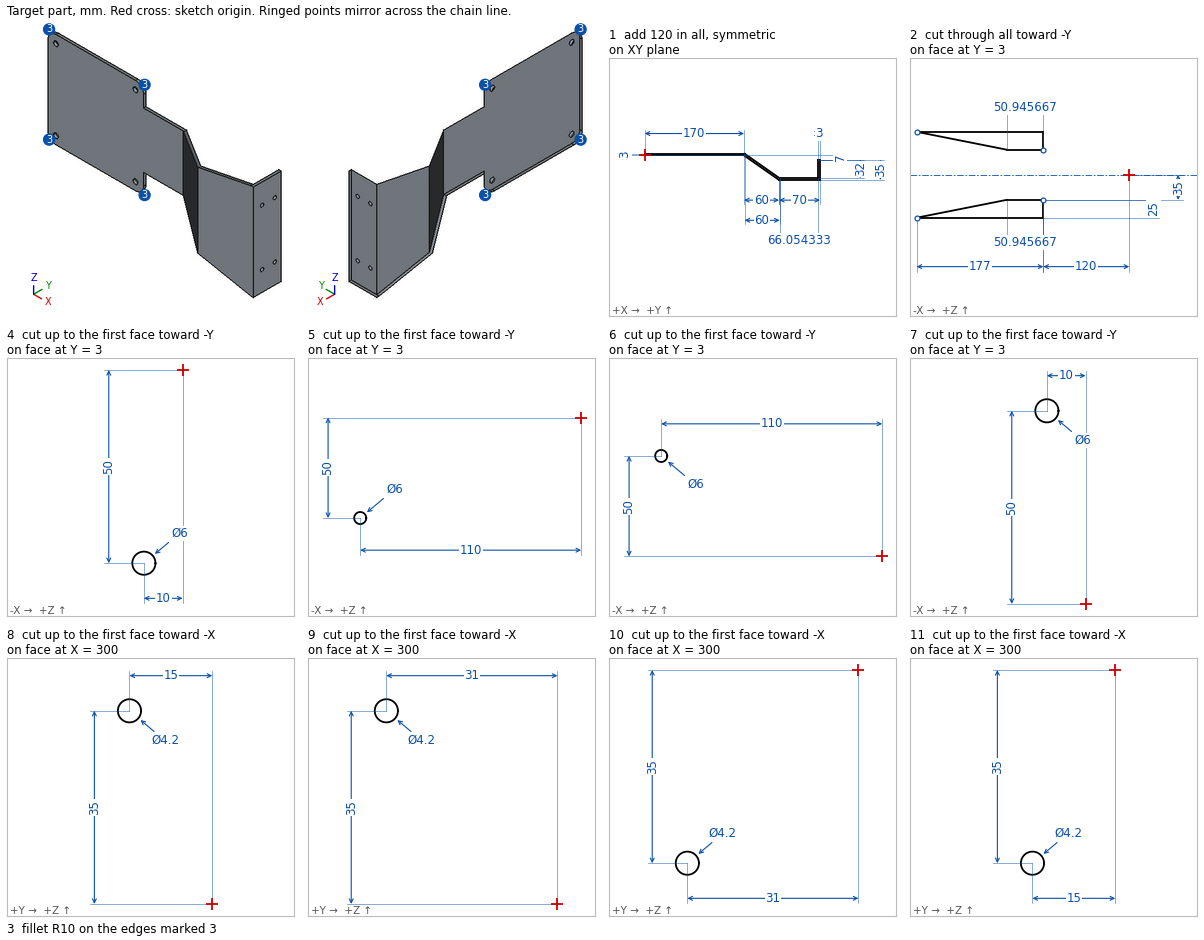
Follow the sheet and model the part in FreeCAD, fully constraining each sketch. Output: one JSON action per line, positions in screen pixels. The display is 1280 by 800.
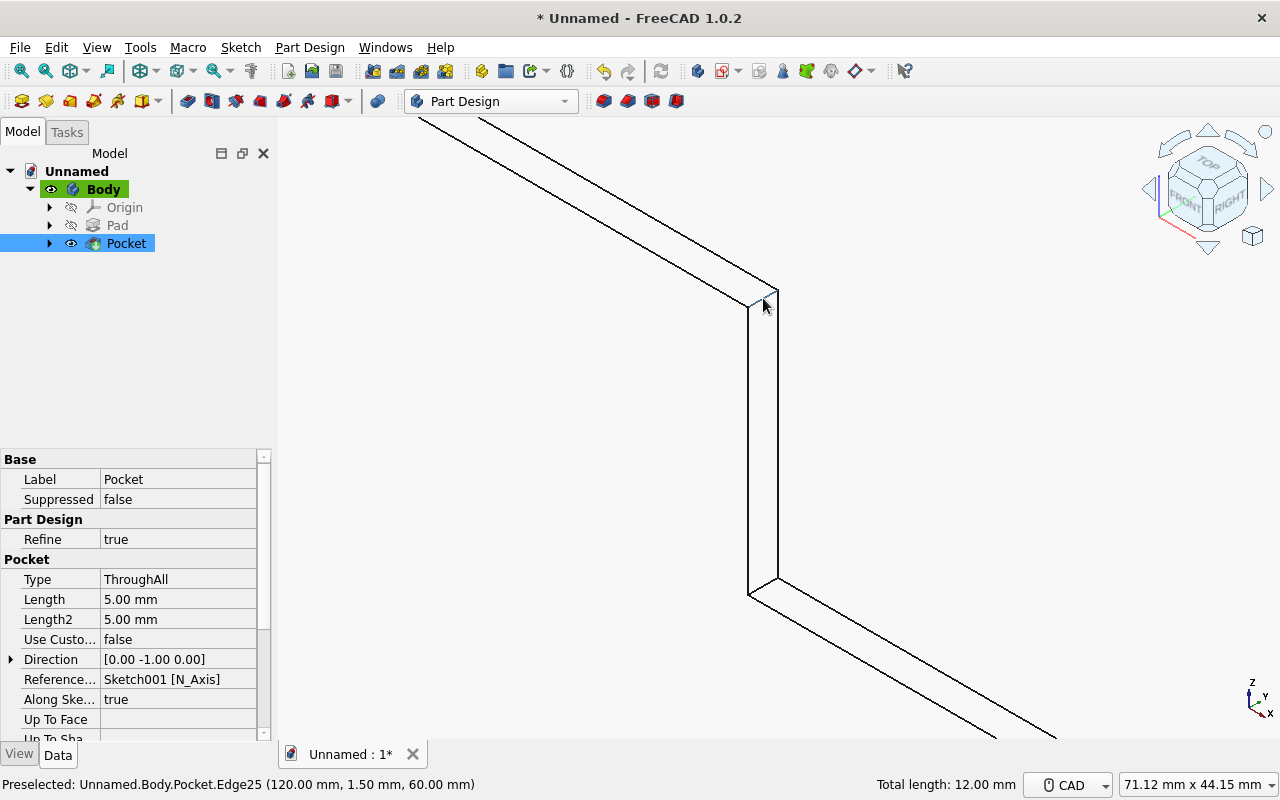
{"action": "key", "text": "v 1"}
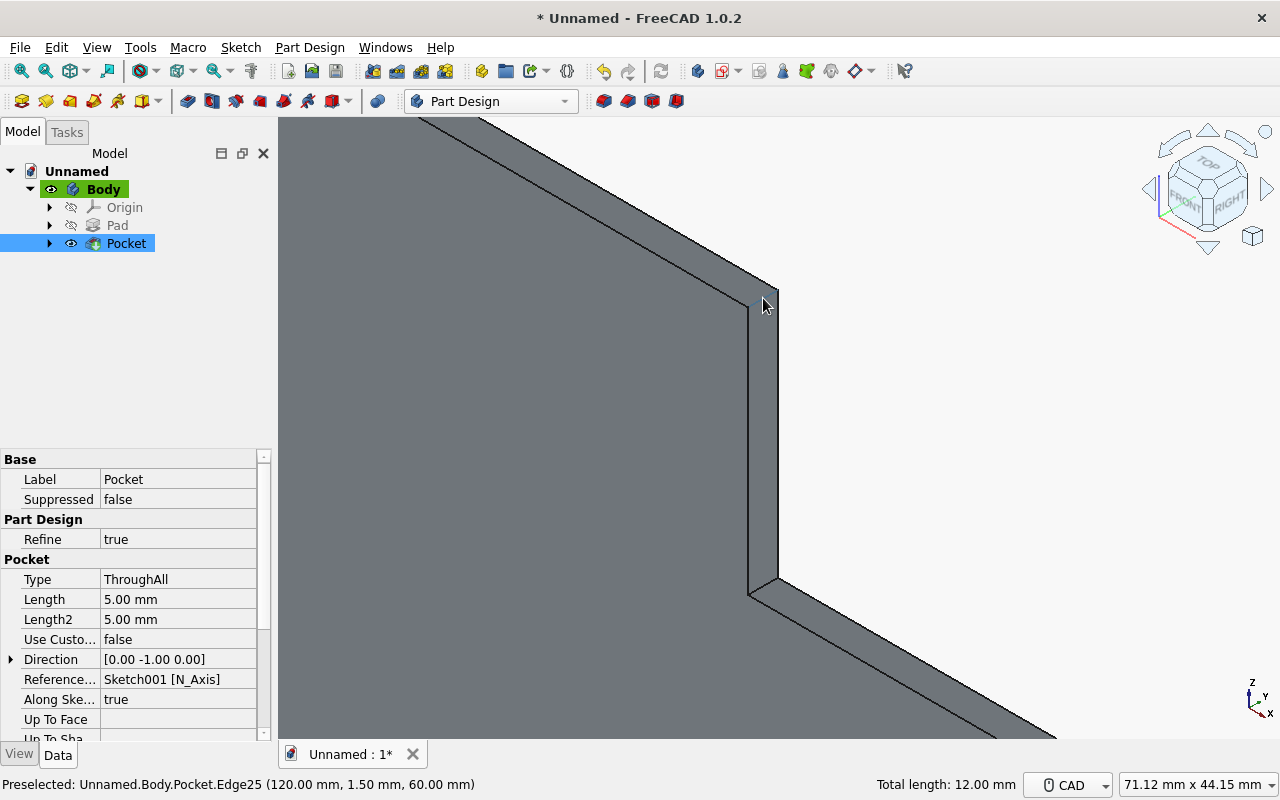
{"action": "left_click", "coordinate": [604, 102]}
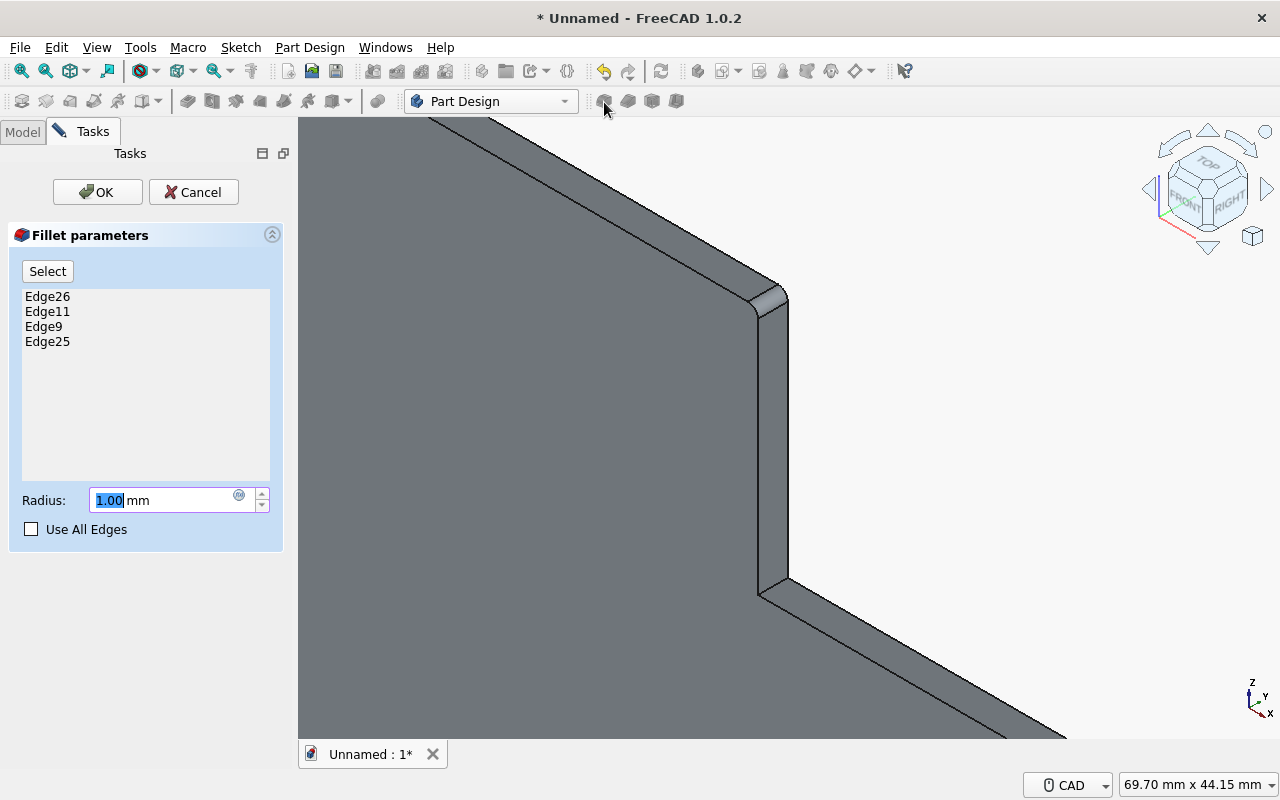
{"action": "type", "text": "10"}
{"action": "key", "text": "Tab"}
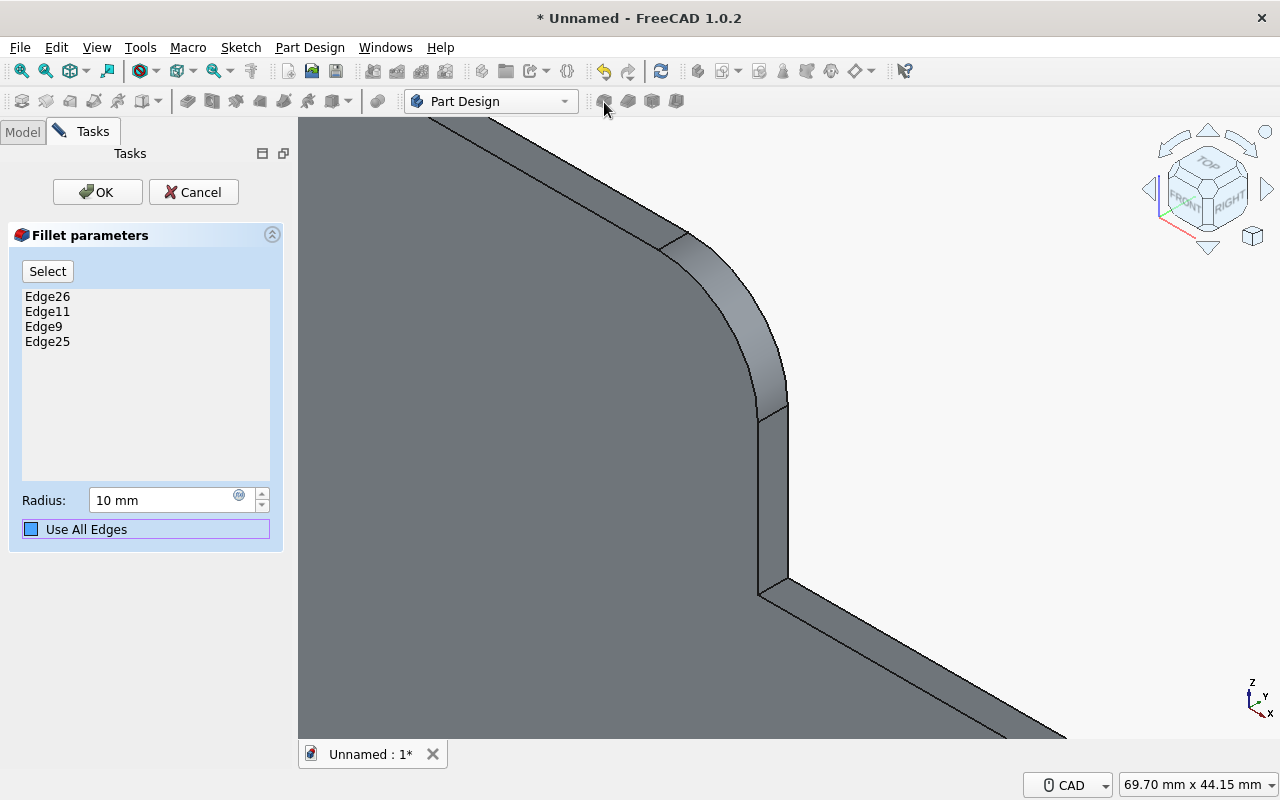
{"action": "left_click", "coordinate": [98, 192]}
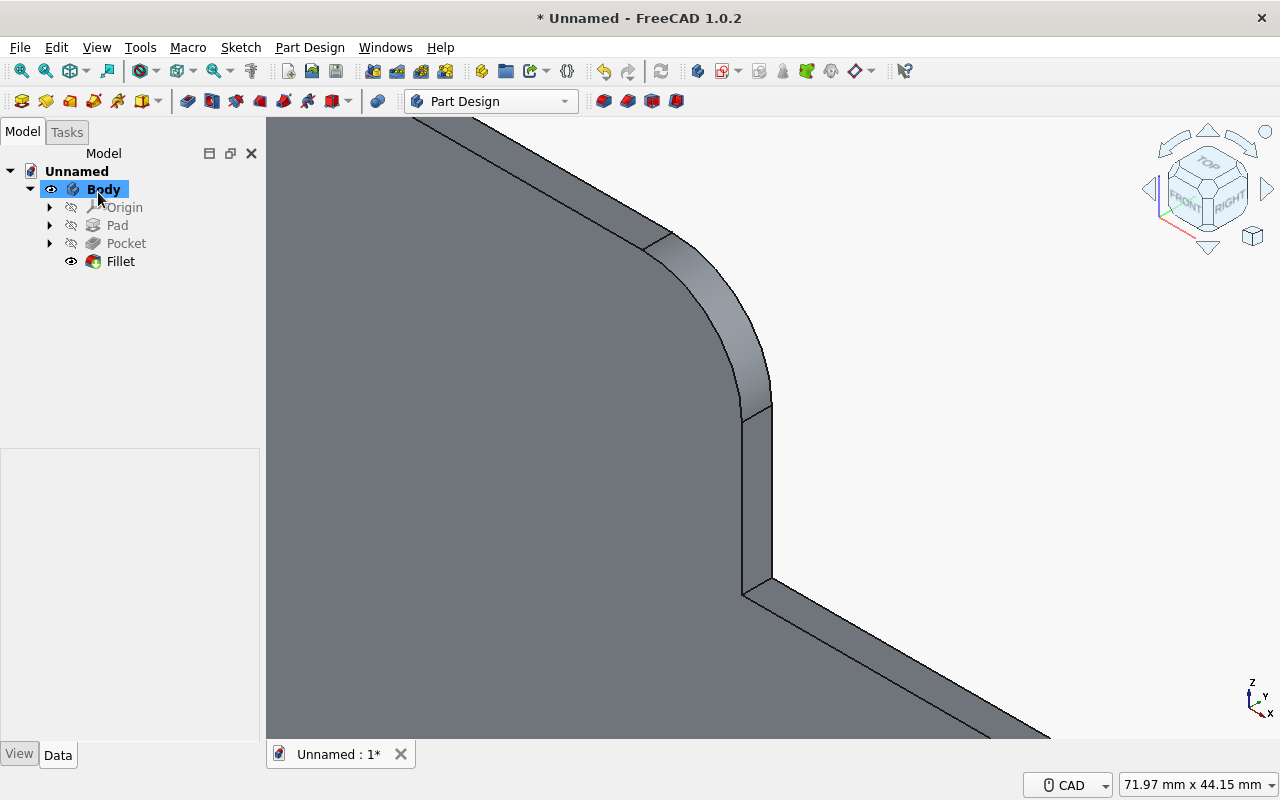
{"action": "left_click", "coordinate": [22, 72]}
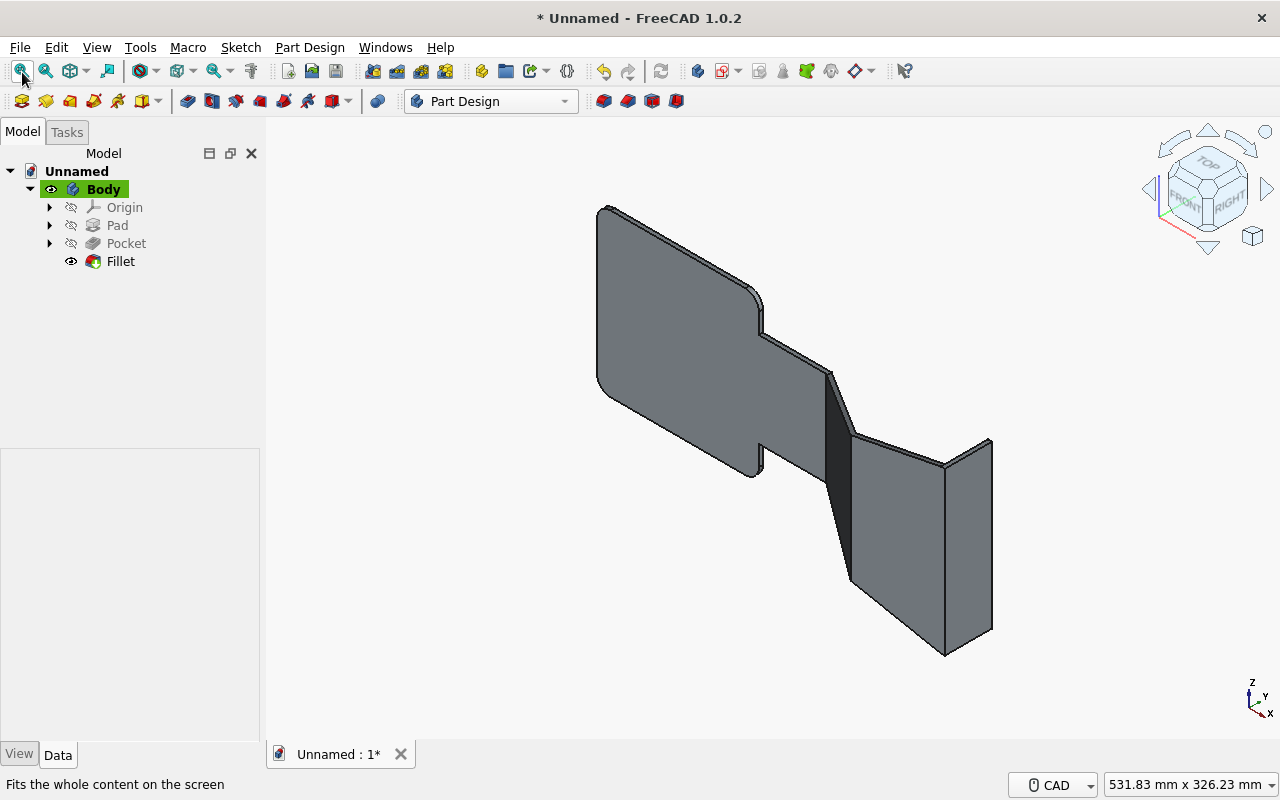
{"action": "key", "text": "4"}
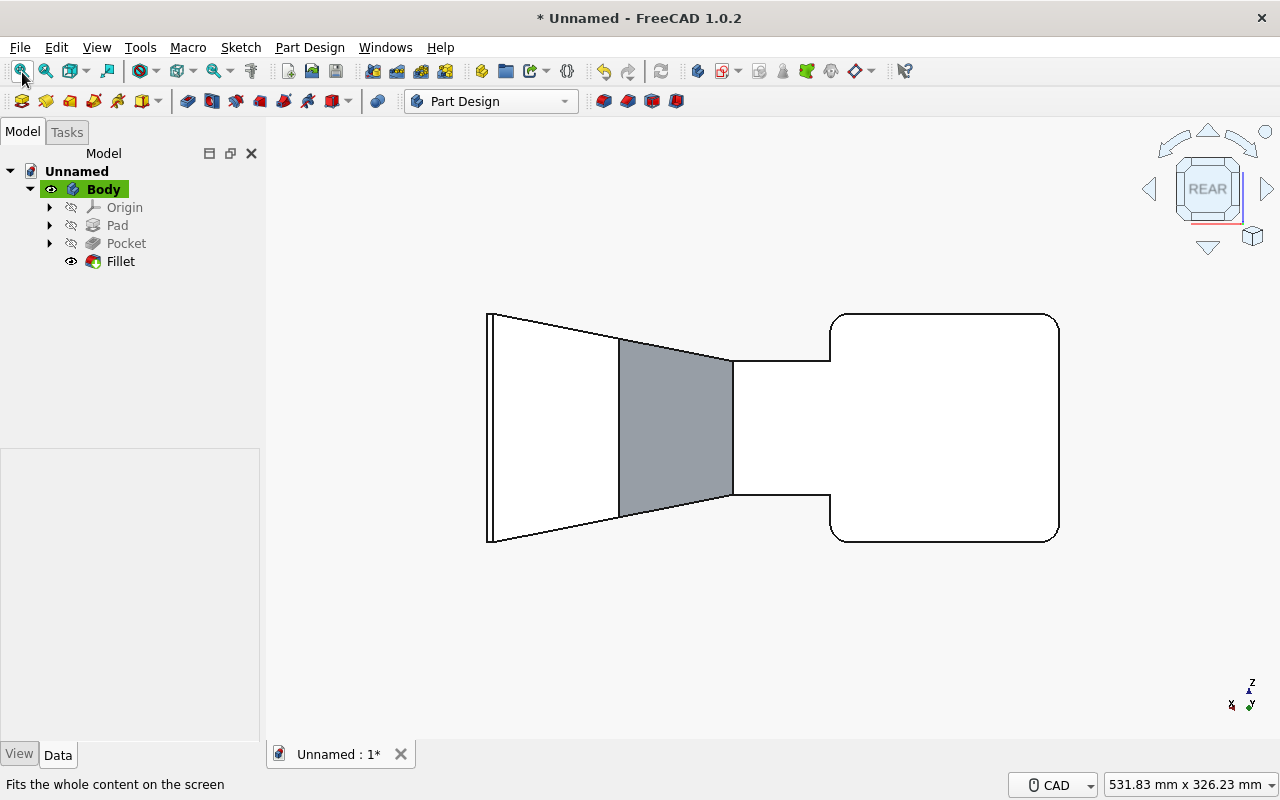
{"action": "left_click", "coordinate": [943, 427]}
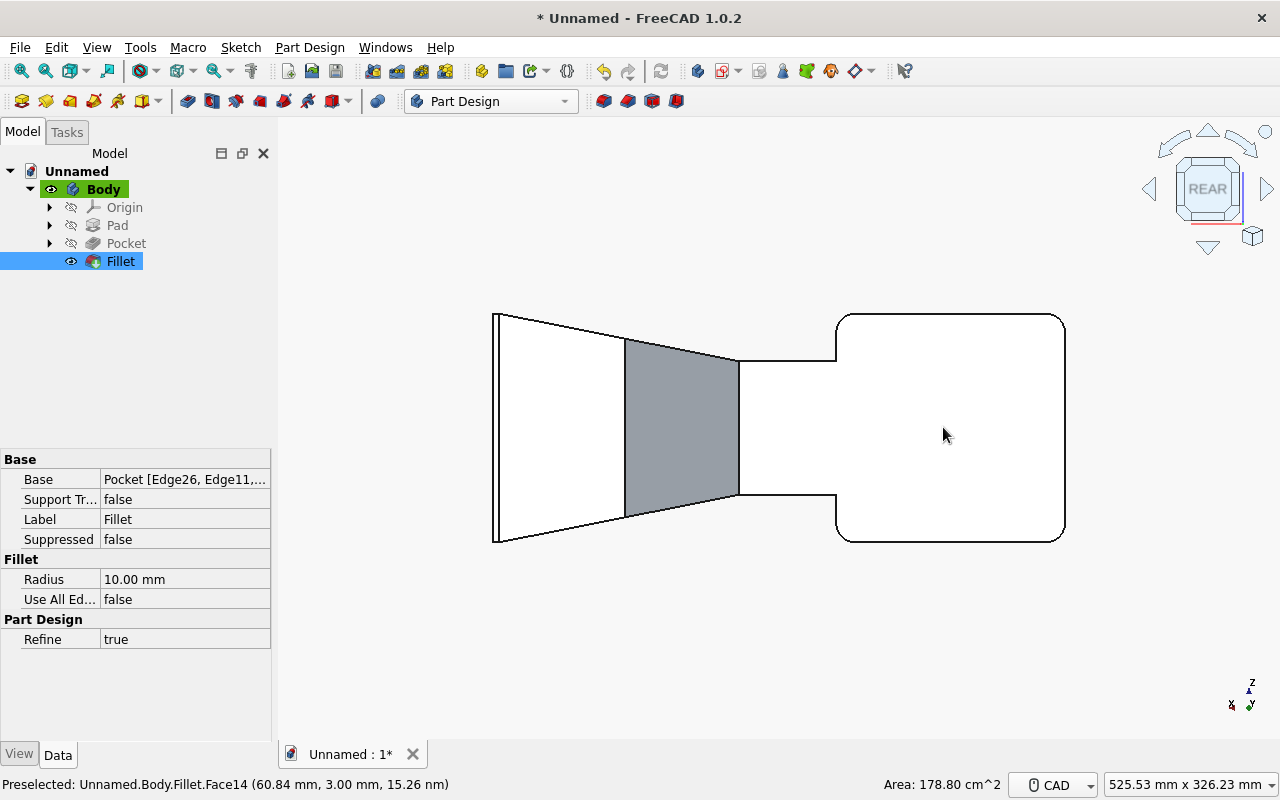
{"action": "left_click", "coordinate": [722, 72]}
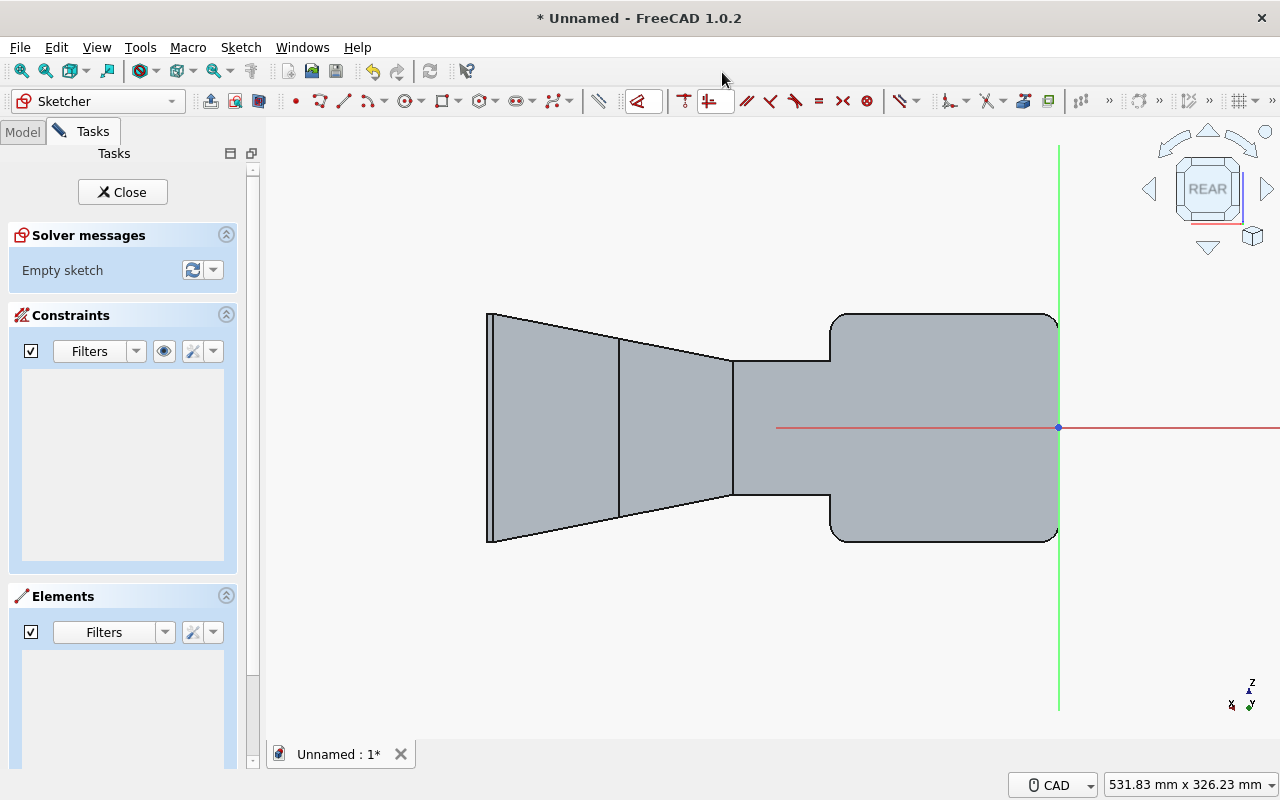
{"action": "scroll", "coordinate": [1058, 528], "scroll_direction": "up", "scroll_amount": 15}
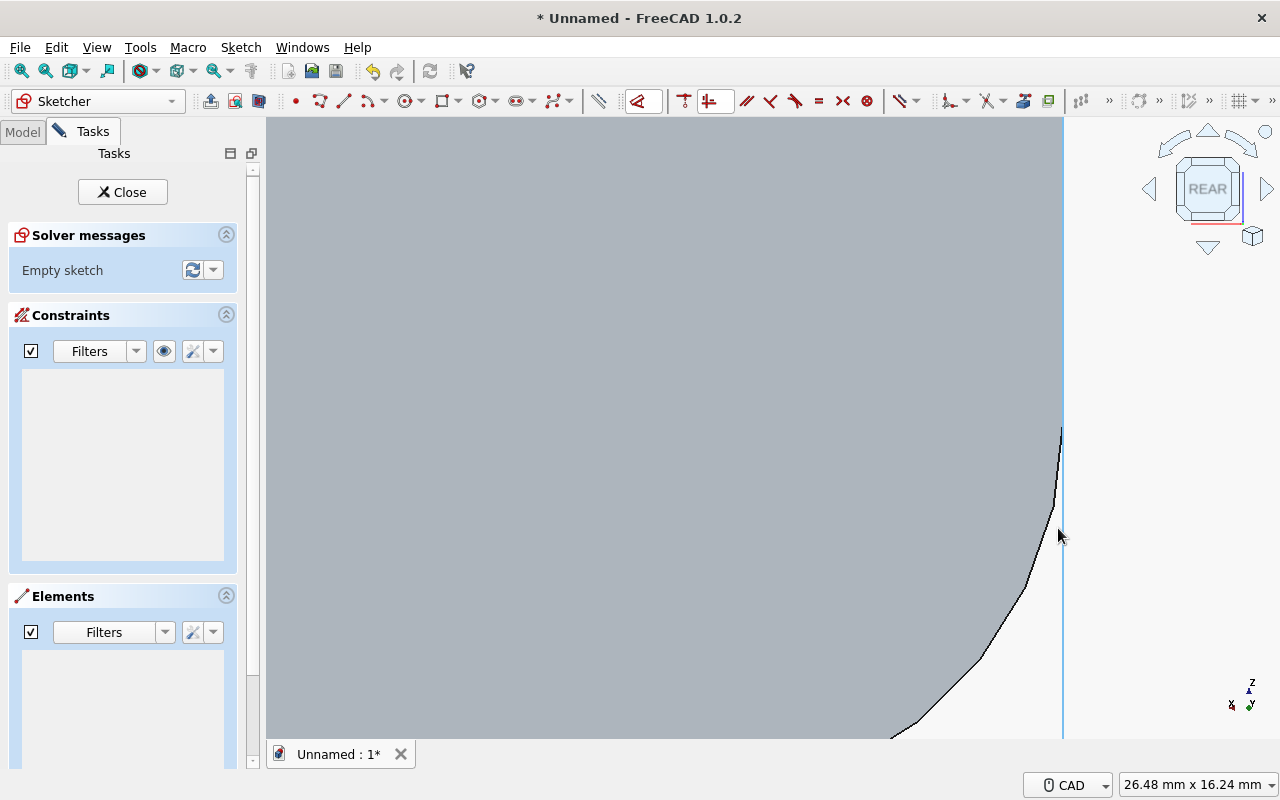
{"action": "scroll", "coordinate": [650, 414], "scroll_direction": "up", "scroll_amount": 3}